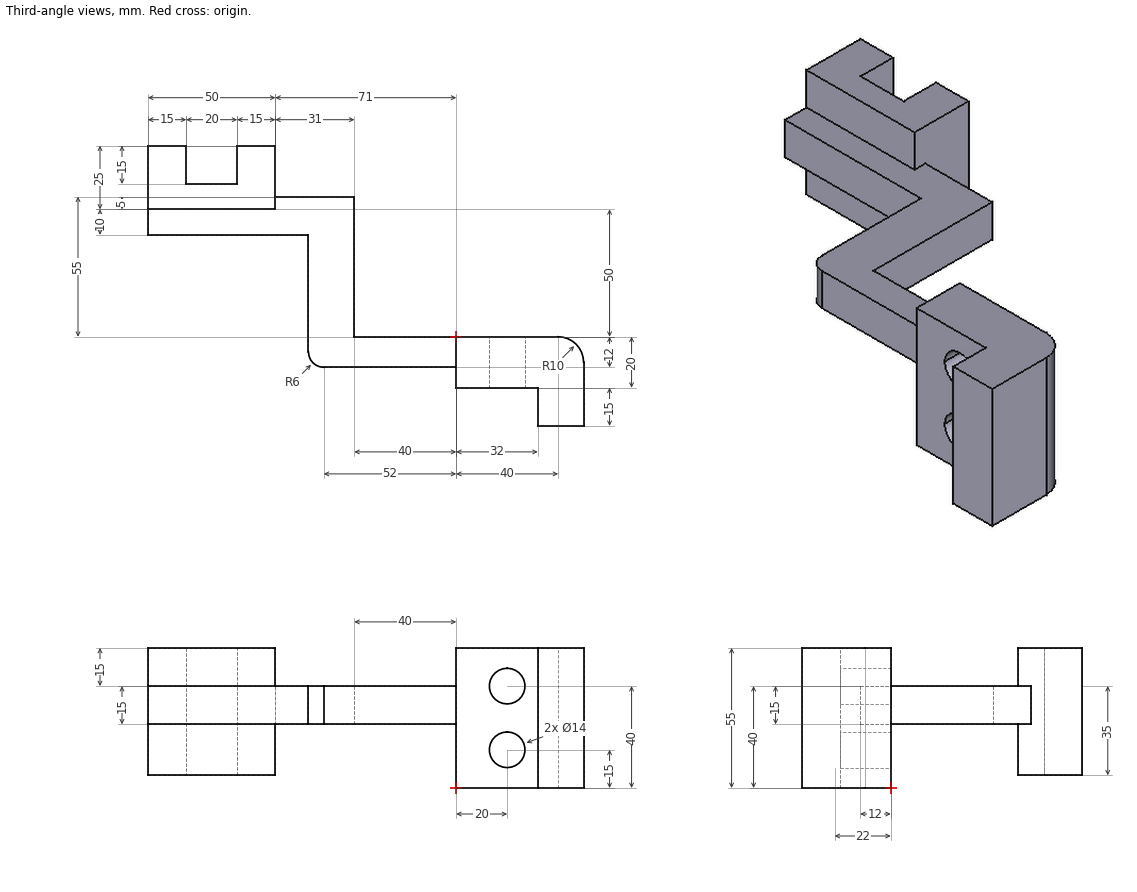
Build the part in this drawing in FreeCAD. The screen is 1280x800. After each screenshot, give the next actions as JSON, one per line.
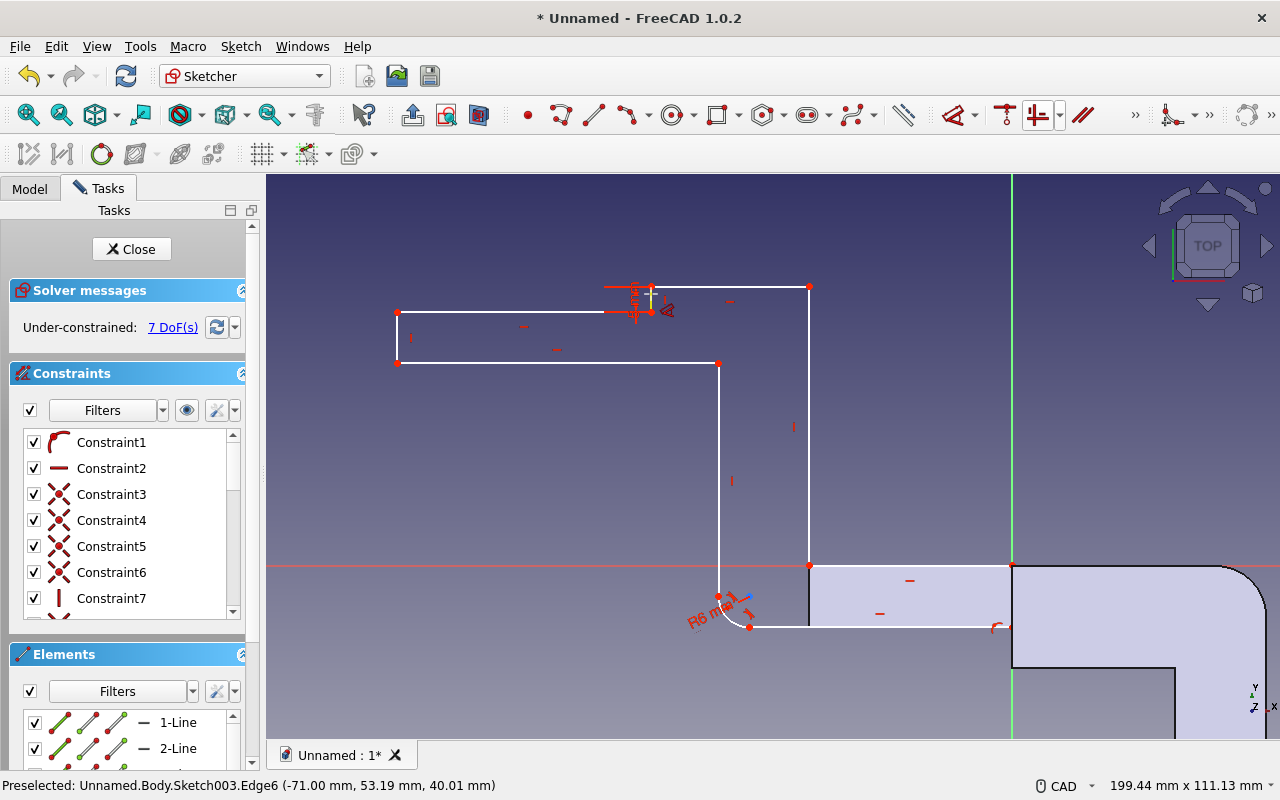
{"action": "left_click", "coordinate": [828, 627]}
{"action": "left_click", "coordinate": [881, 661]}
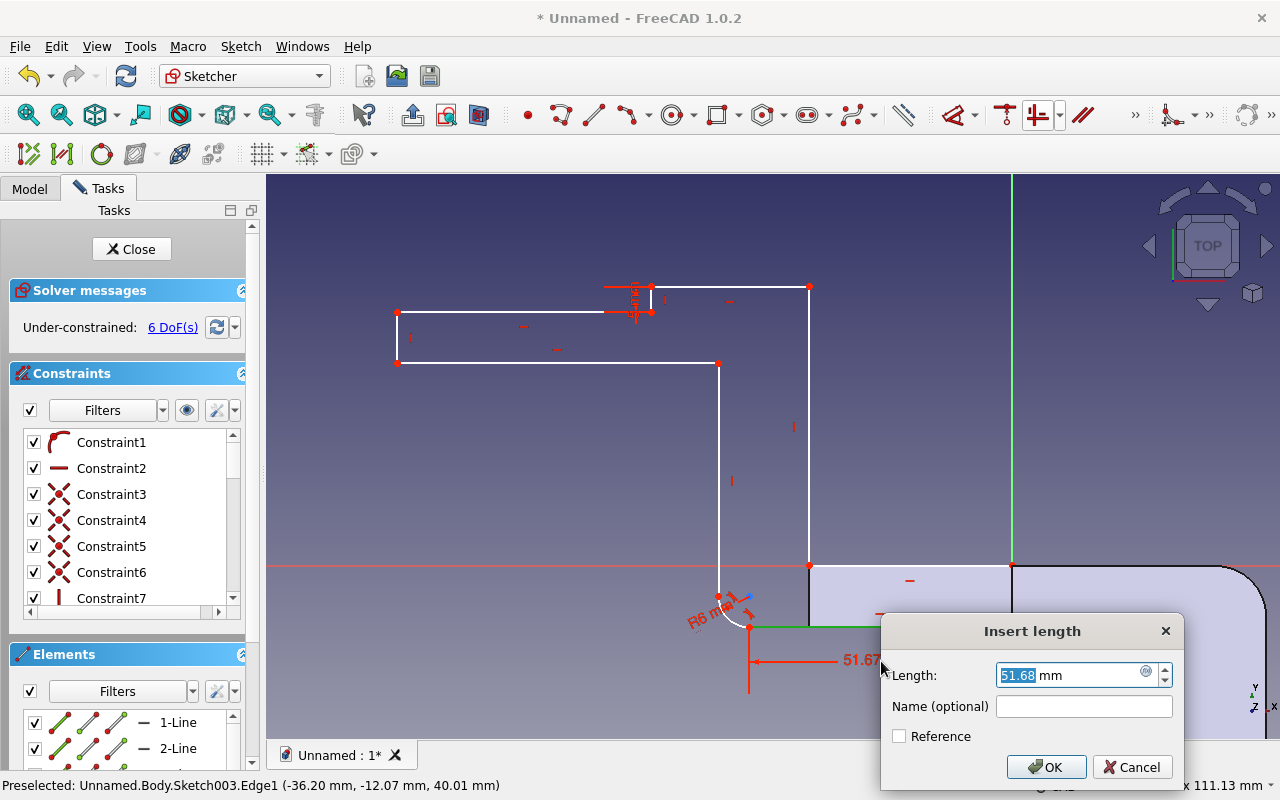
{"action": "type", "text": "52"}
{"action": "key", "text": "Return"}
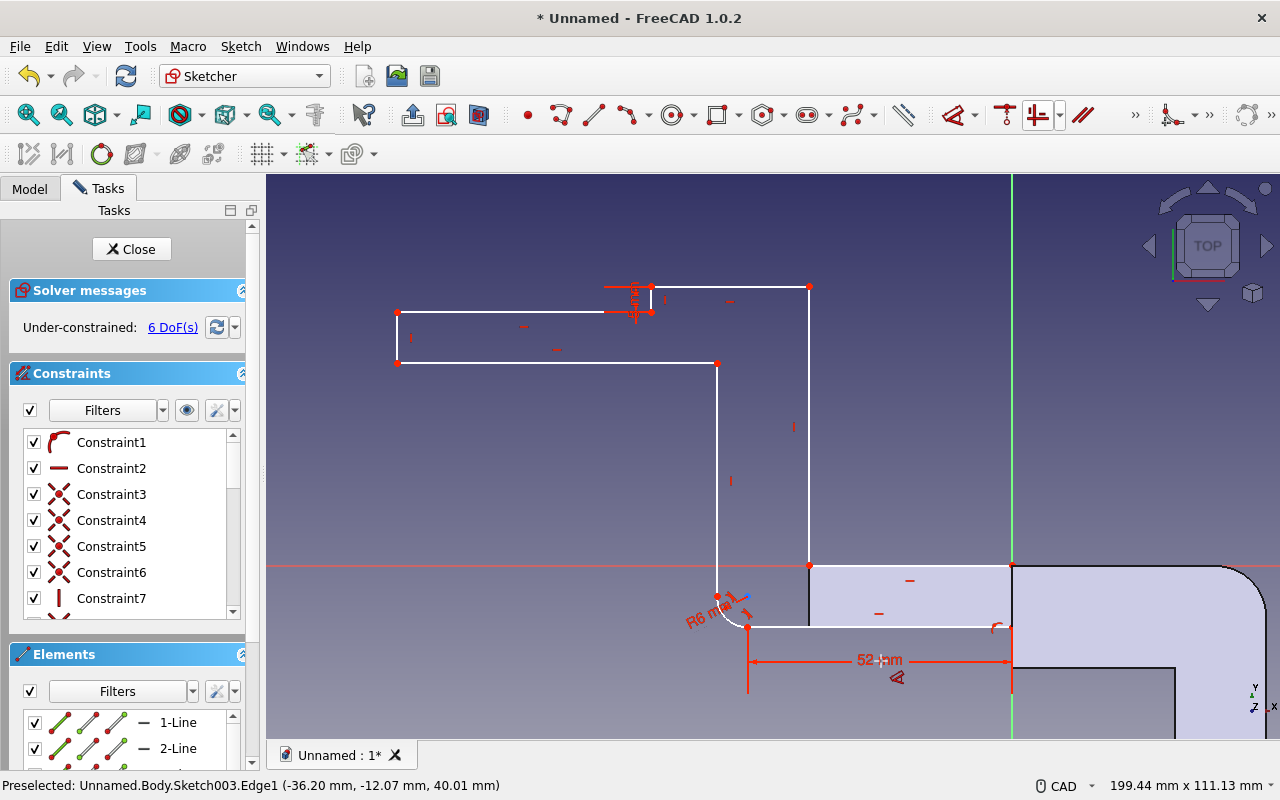
{"action": "left_click", "coordinate": [1012, 609]}
{"action": "left_click", "coordinate": [1046, 597]}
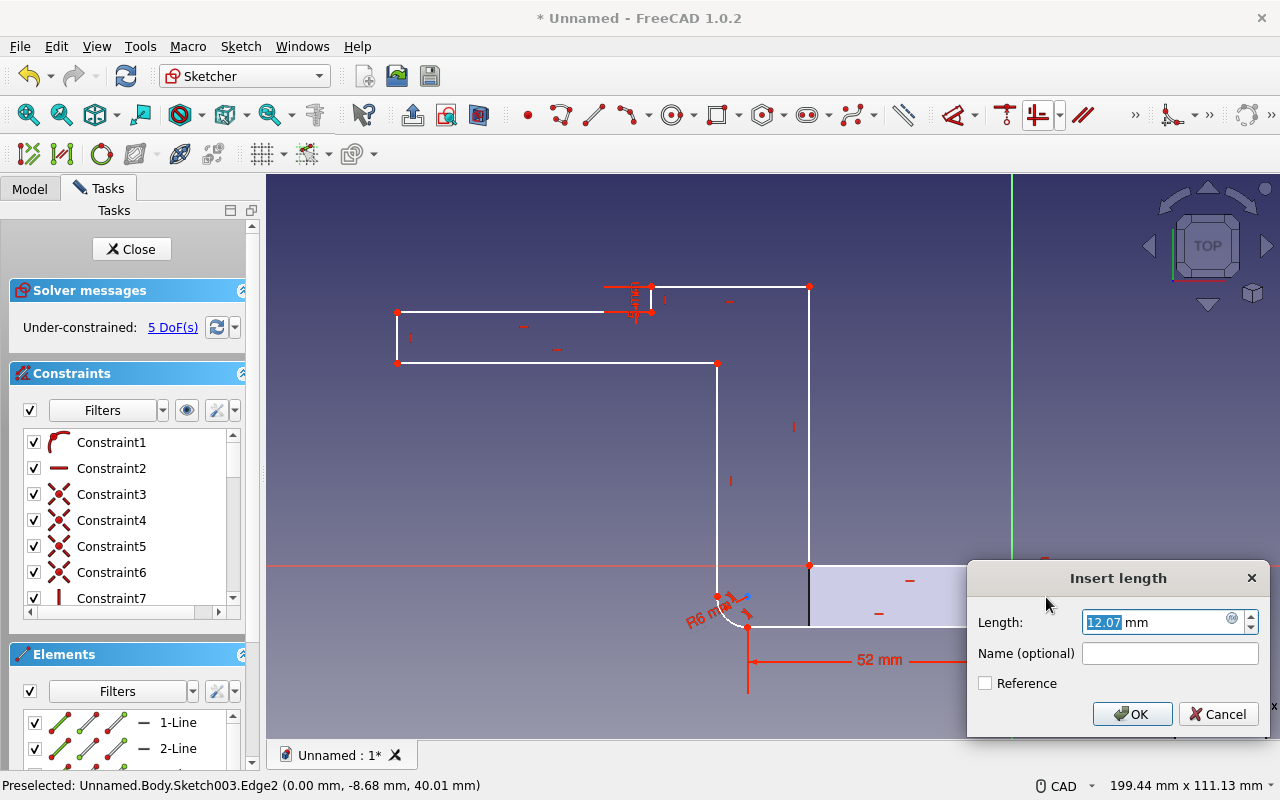
{"action": "type", "text": "12"}
{"action": "key", "text": "Return"}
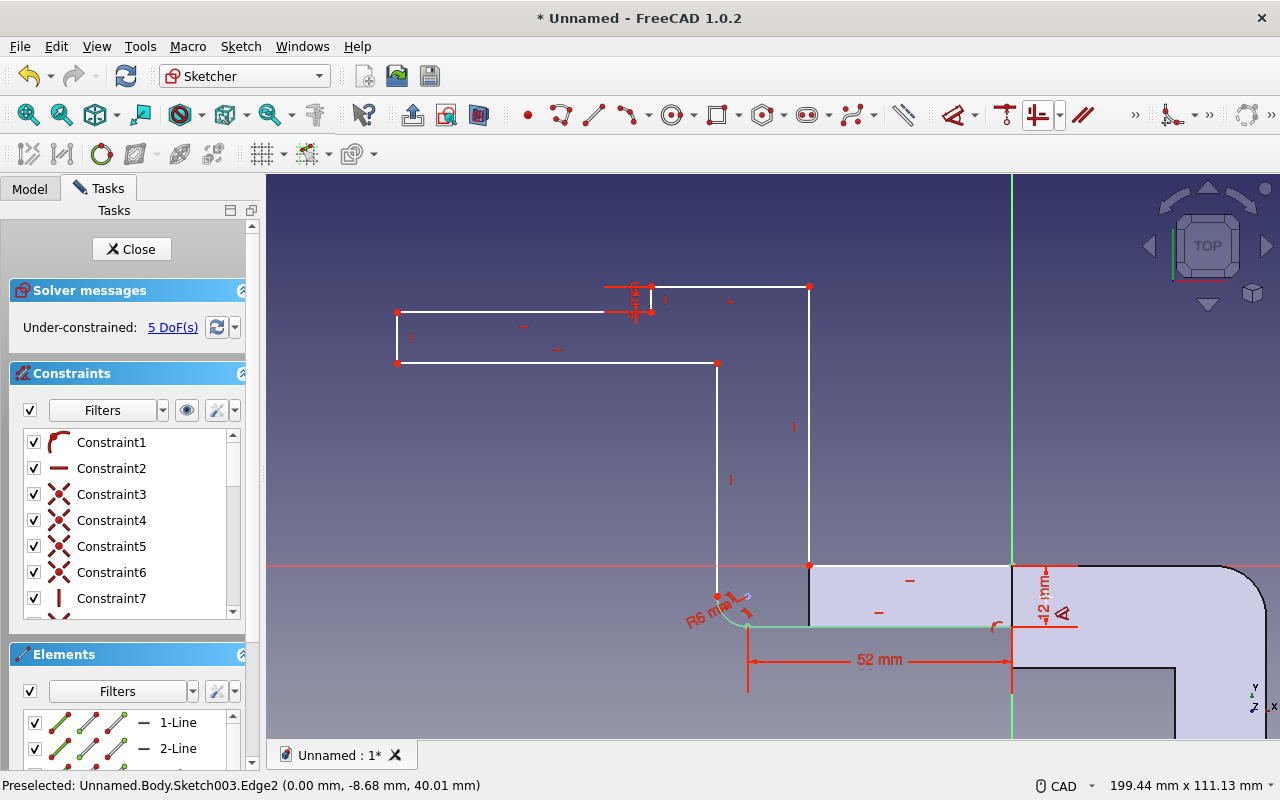
{"action": "left_click", "coordinate": [951, 566]}
{"action": "left_click", "coordinate": [911, 600]}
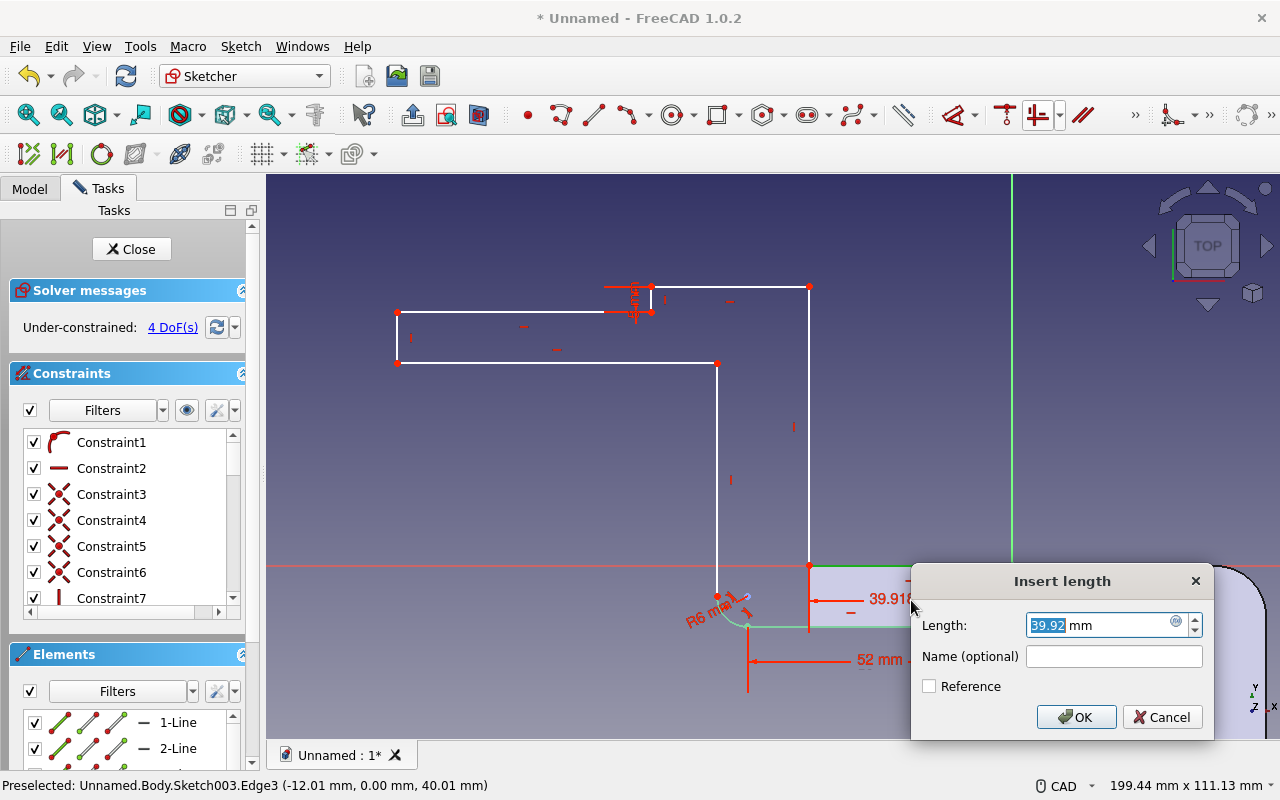
{"action": "type", "text": "40"}
{"action": "key", "text": "Return"}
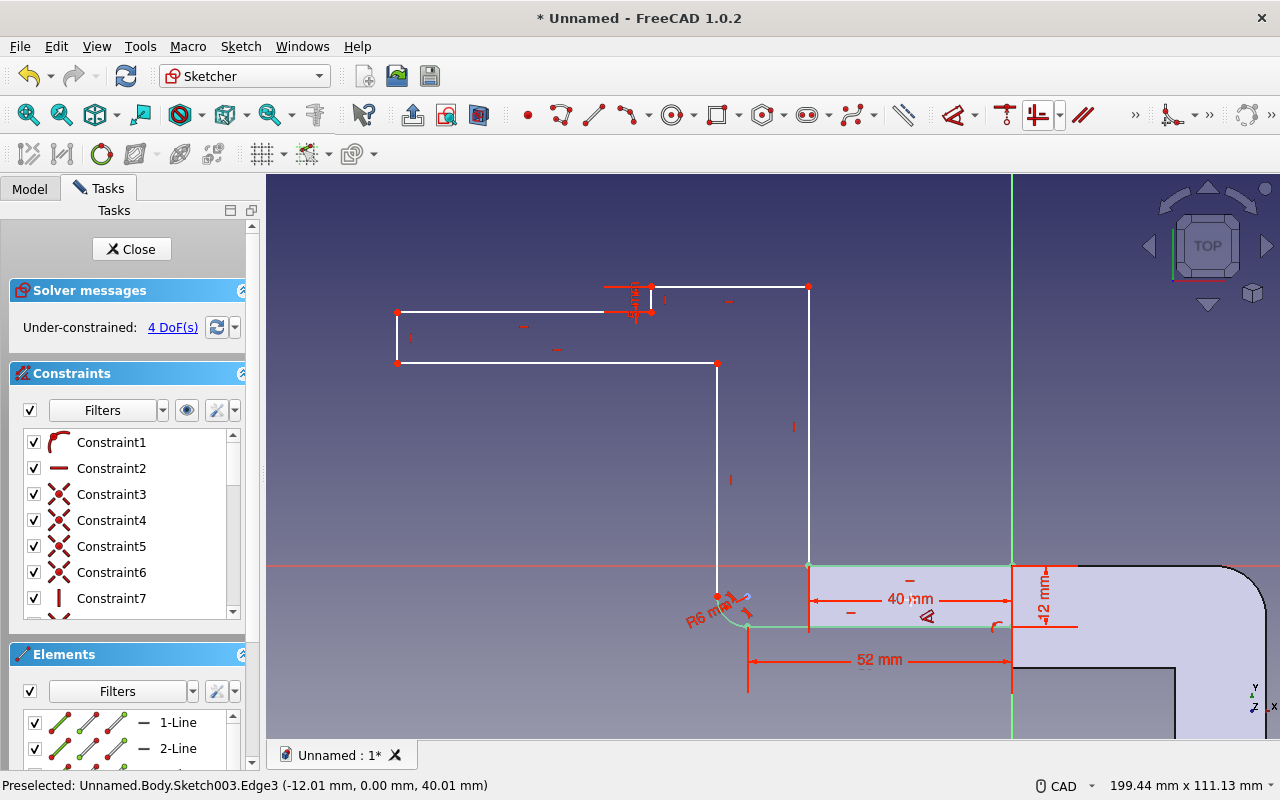
{"action": "left_click", "coordinate": [809, 482]}
{"action": "left_click", "coordinate": [843, 426]}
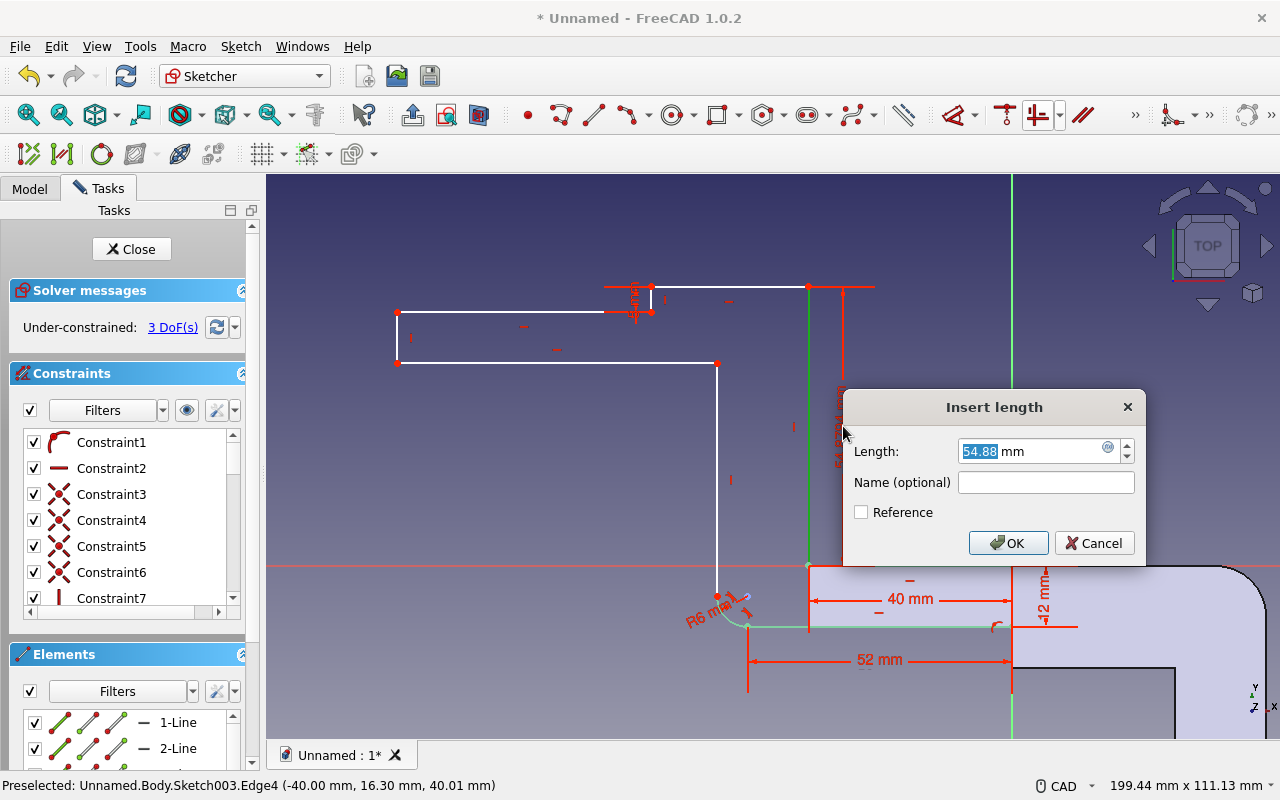
{"action": "type", "text": "55"}
{"action": "key", "text": "Return"}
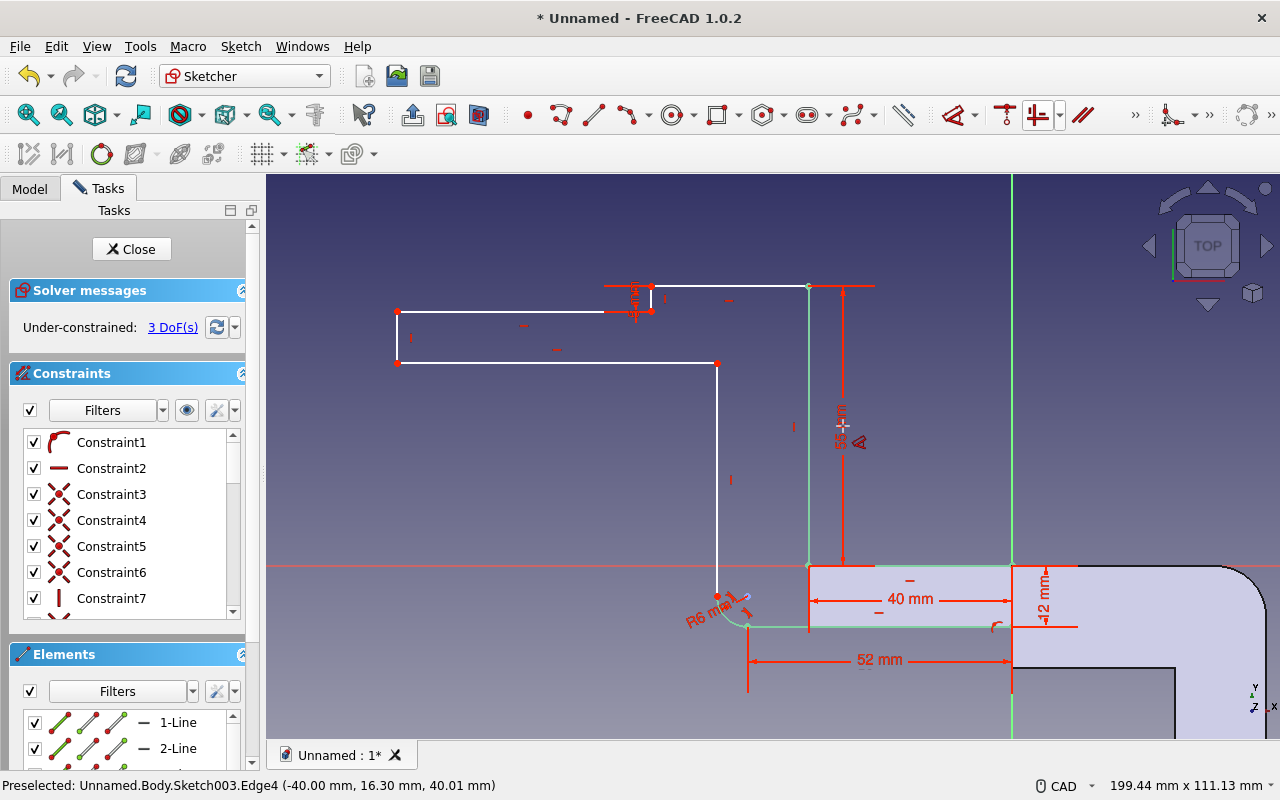
{"action": "left_click", "coordinate": [761, 286]}
{"action": "left_click", "coordinate": [730, 252]}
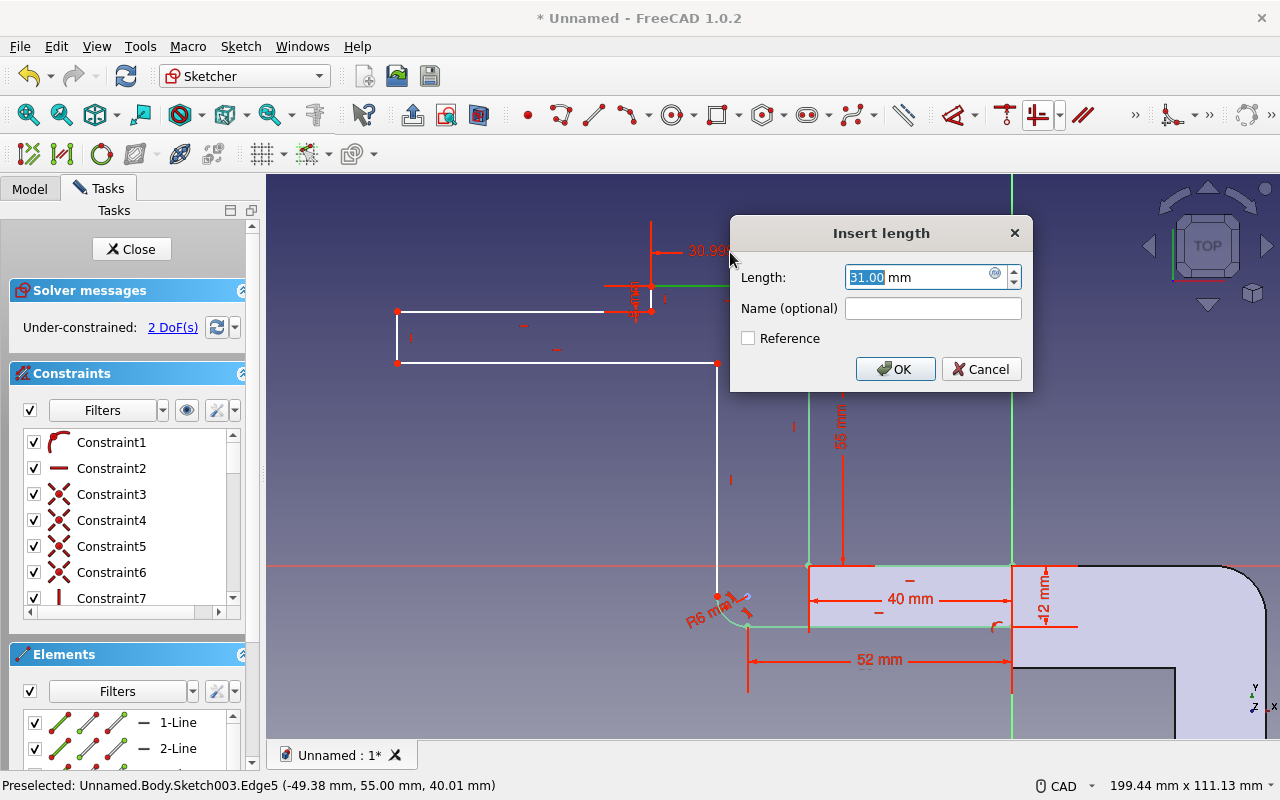
{"action": "type", "text": "31"}
{"action": "key", "text": "Return"}